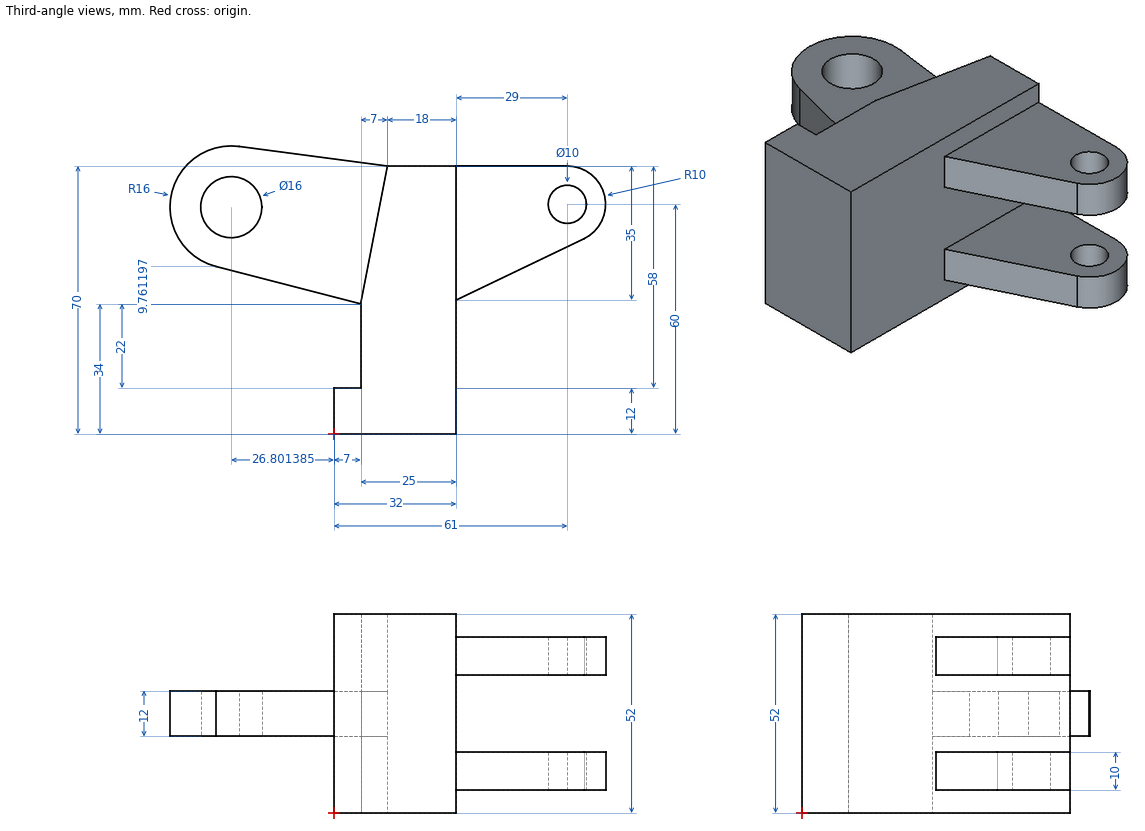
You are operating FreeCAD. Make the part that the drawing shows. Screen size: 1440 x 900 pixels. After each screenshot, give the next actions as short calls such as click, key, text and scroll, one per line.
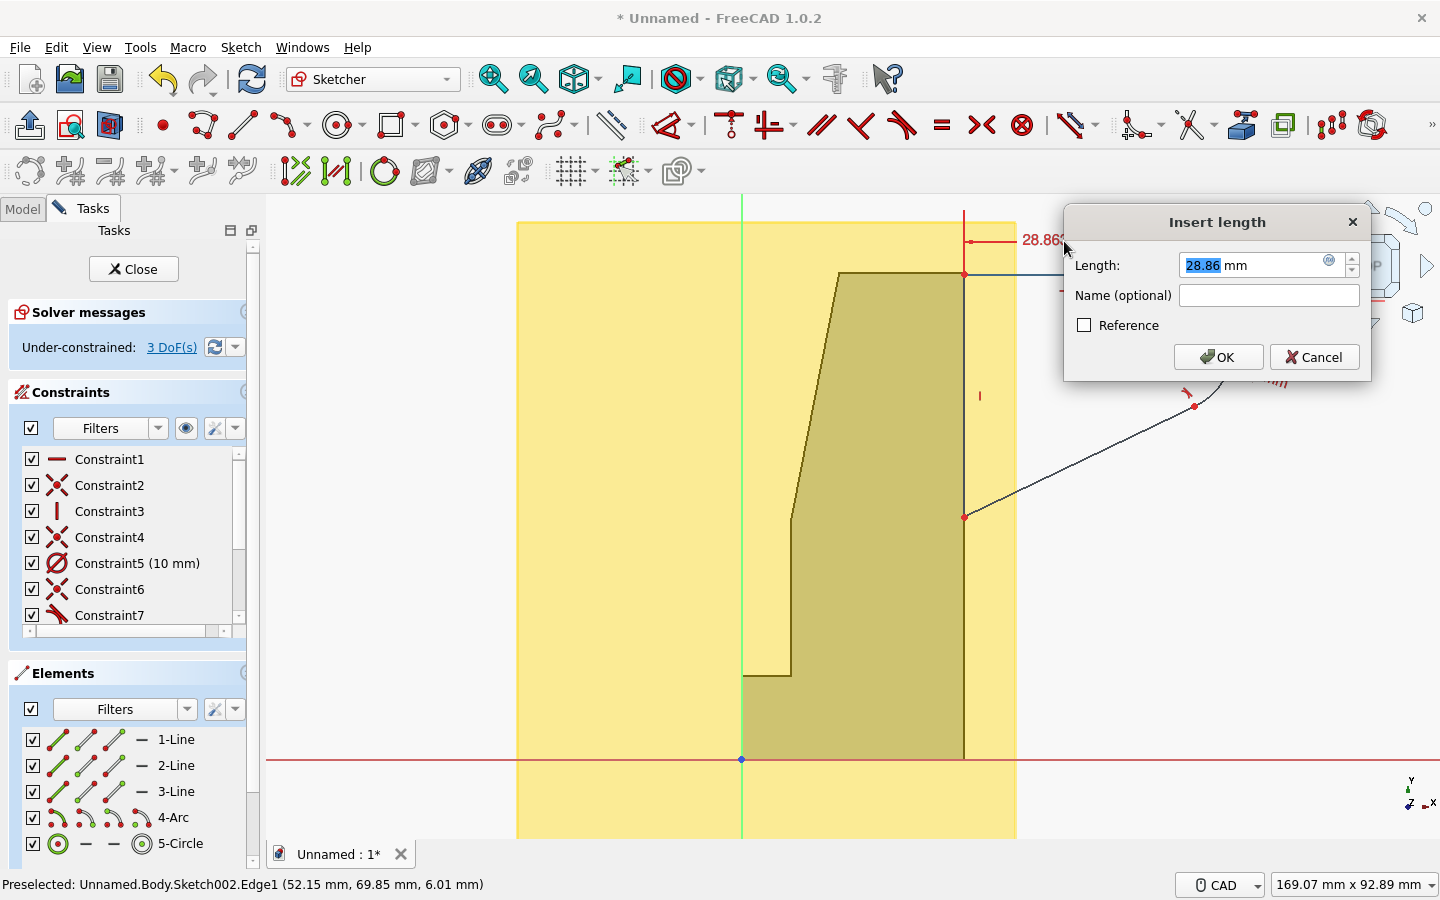
text(29)
key(Return)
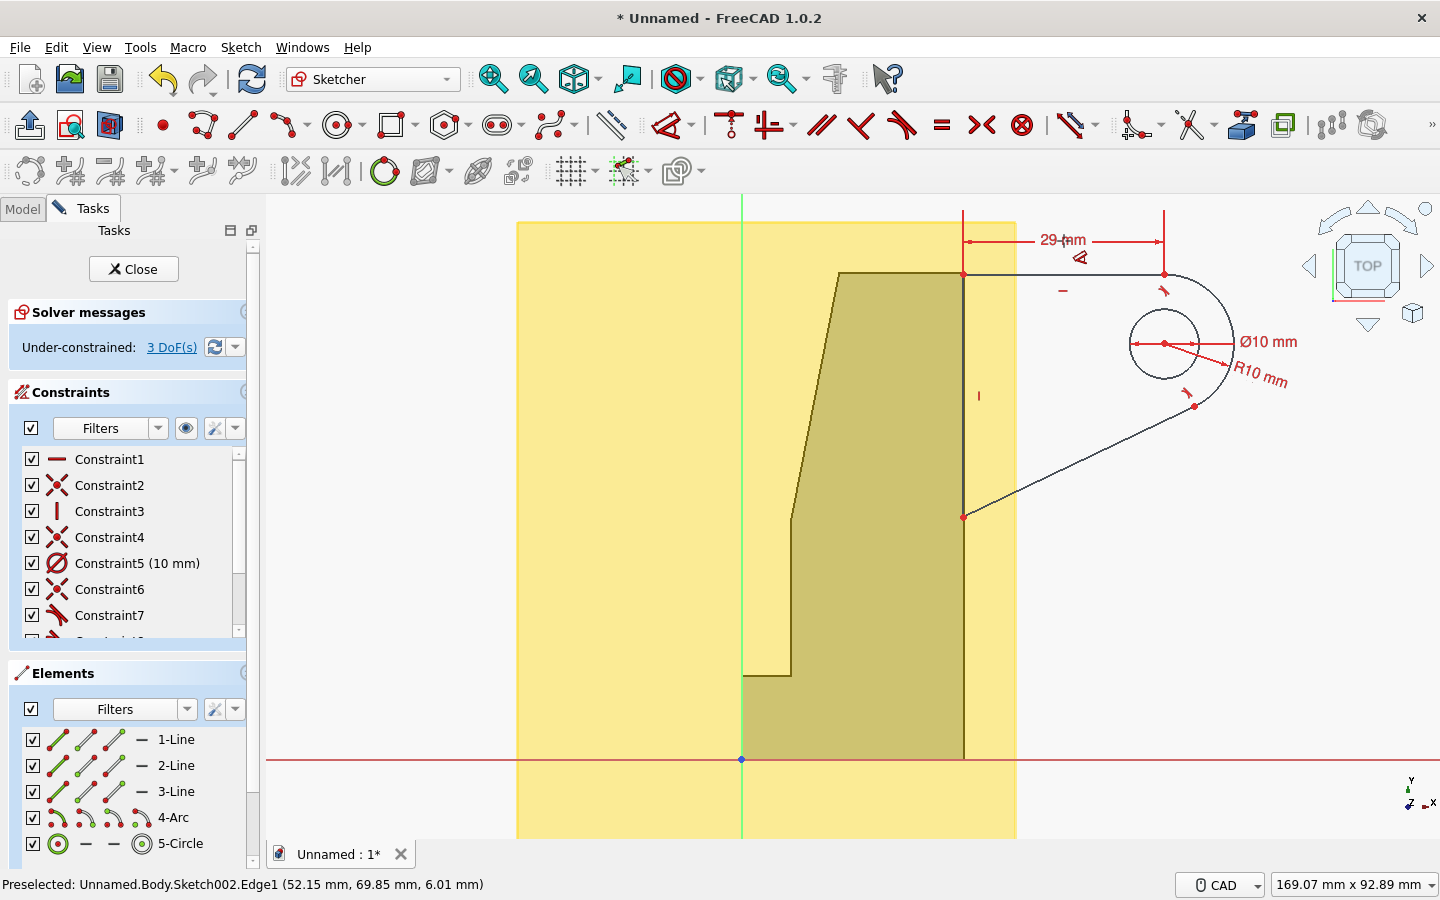
click(963, 347)
click(929, 396)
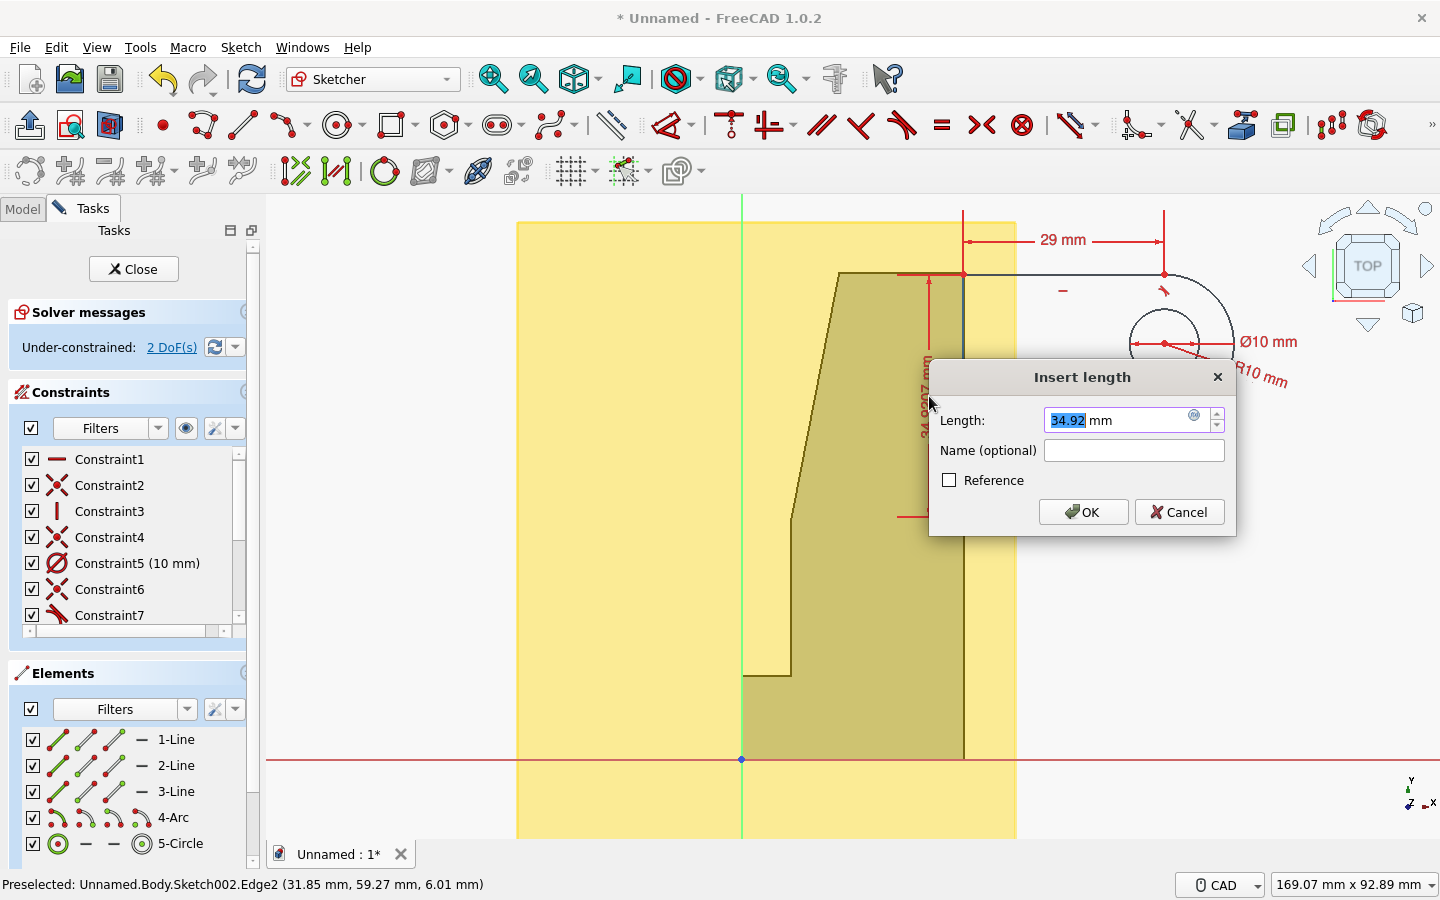
text(35)
key(Return)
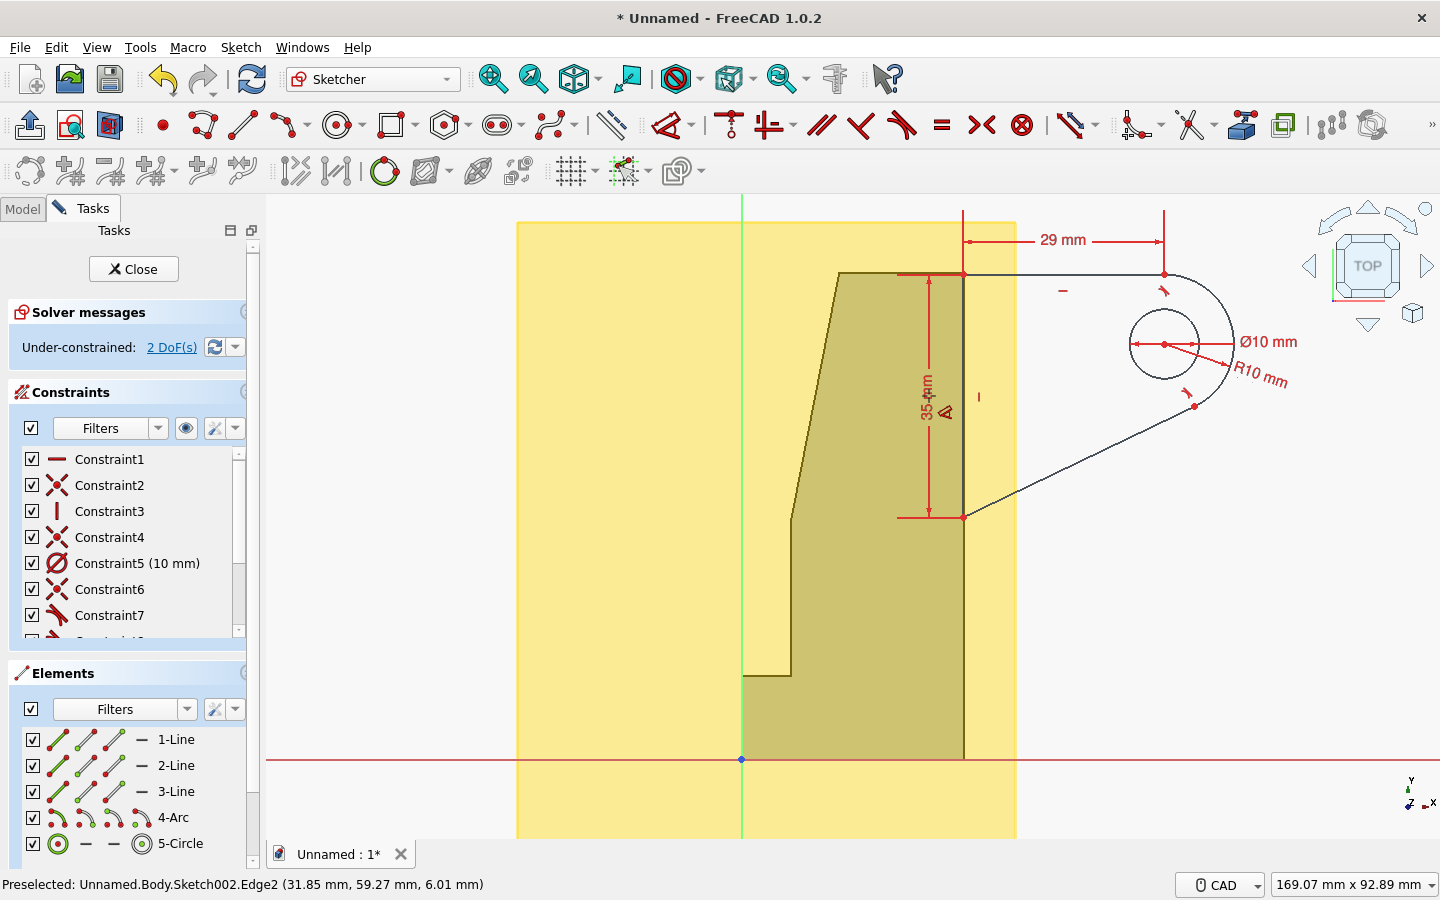
click(1164, 344)
click(953, 794)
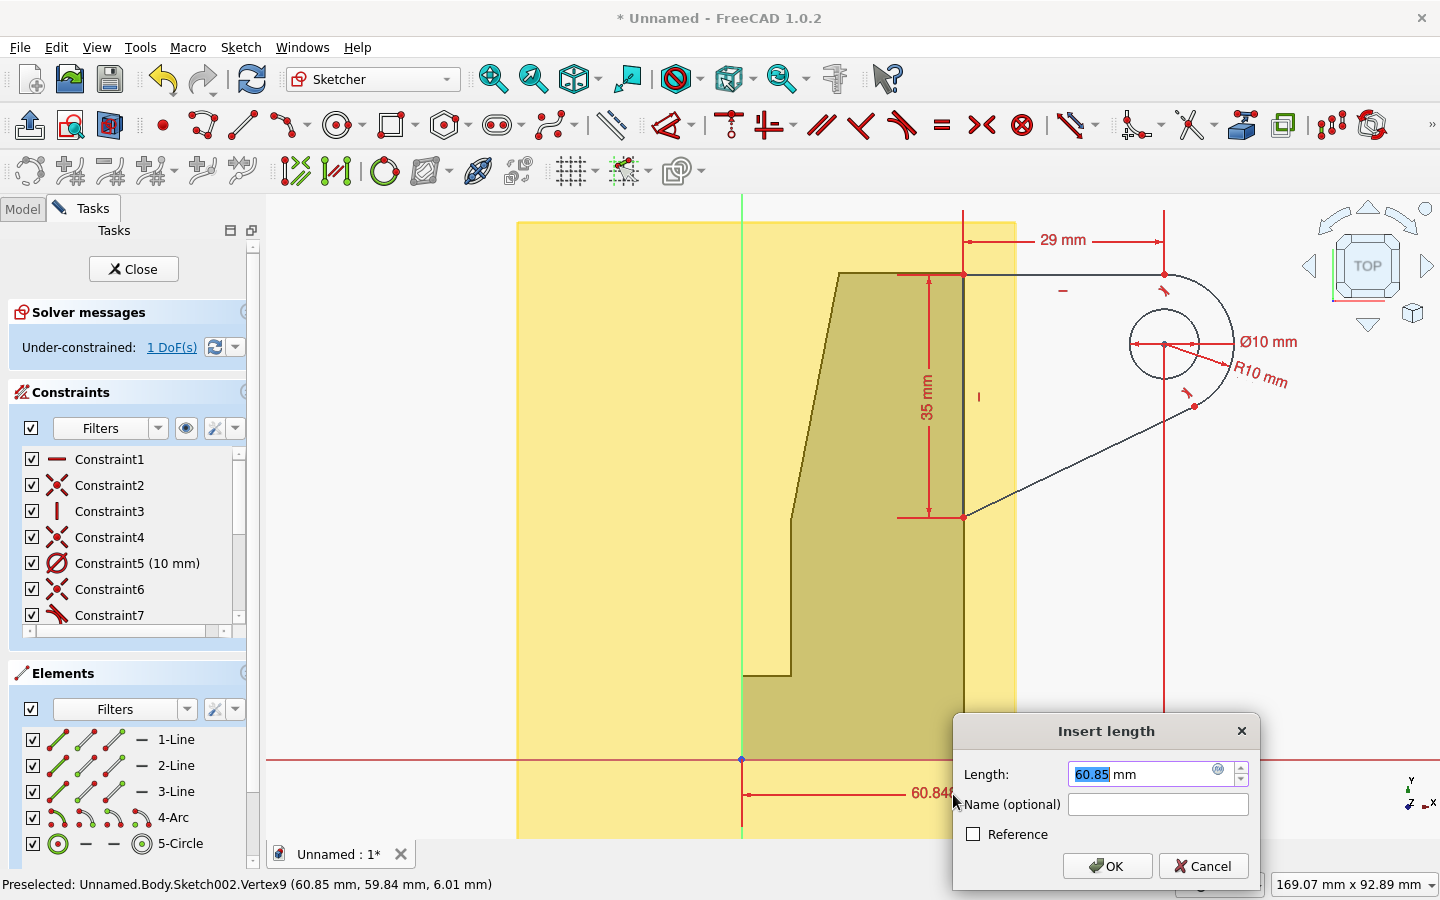
text(61)
key(Return)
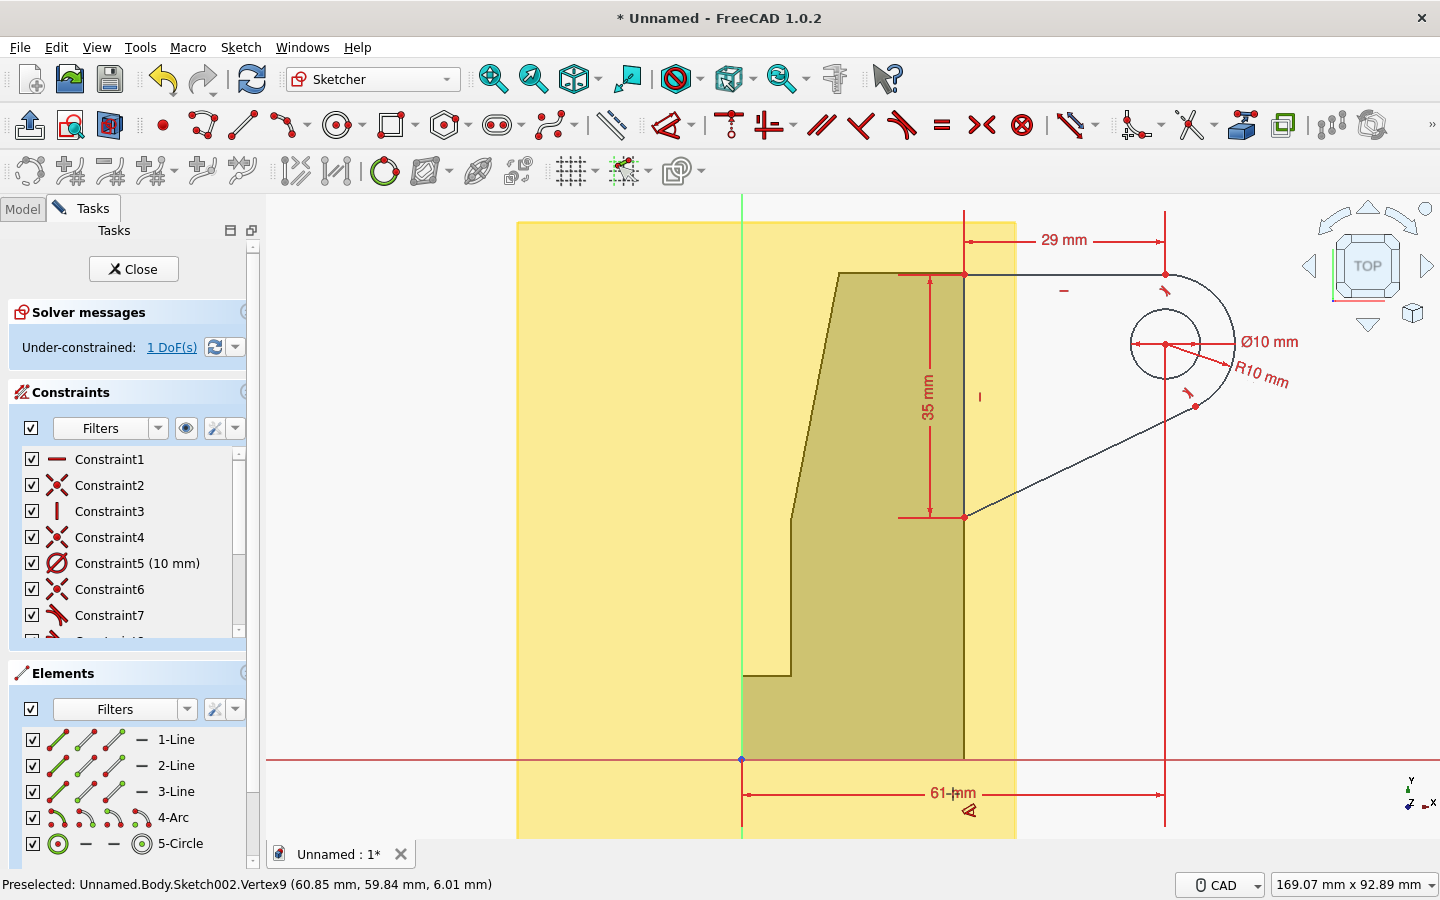
click(1165, 344)
click(708, 552)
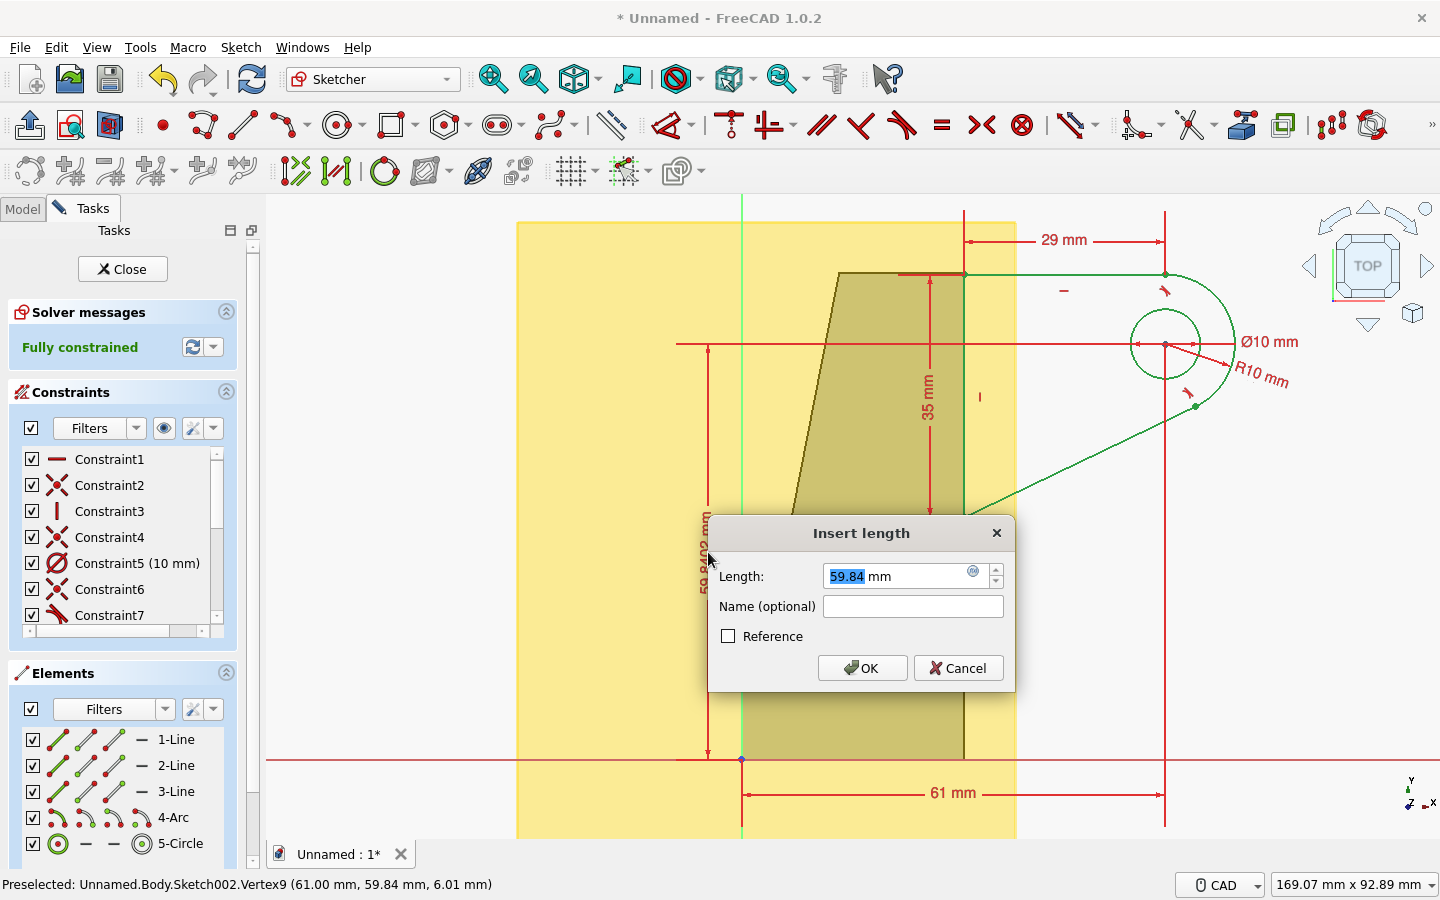
text(60)
key(Return)
key(Escape)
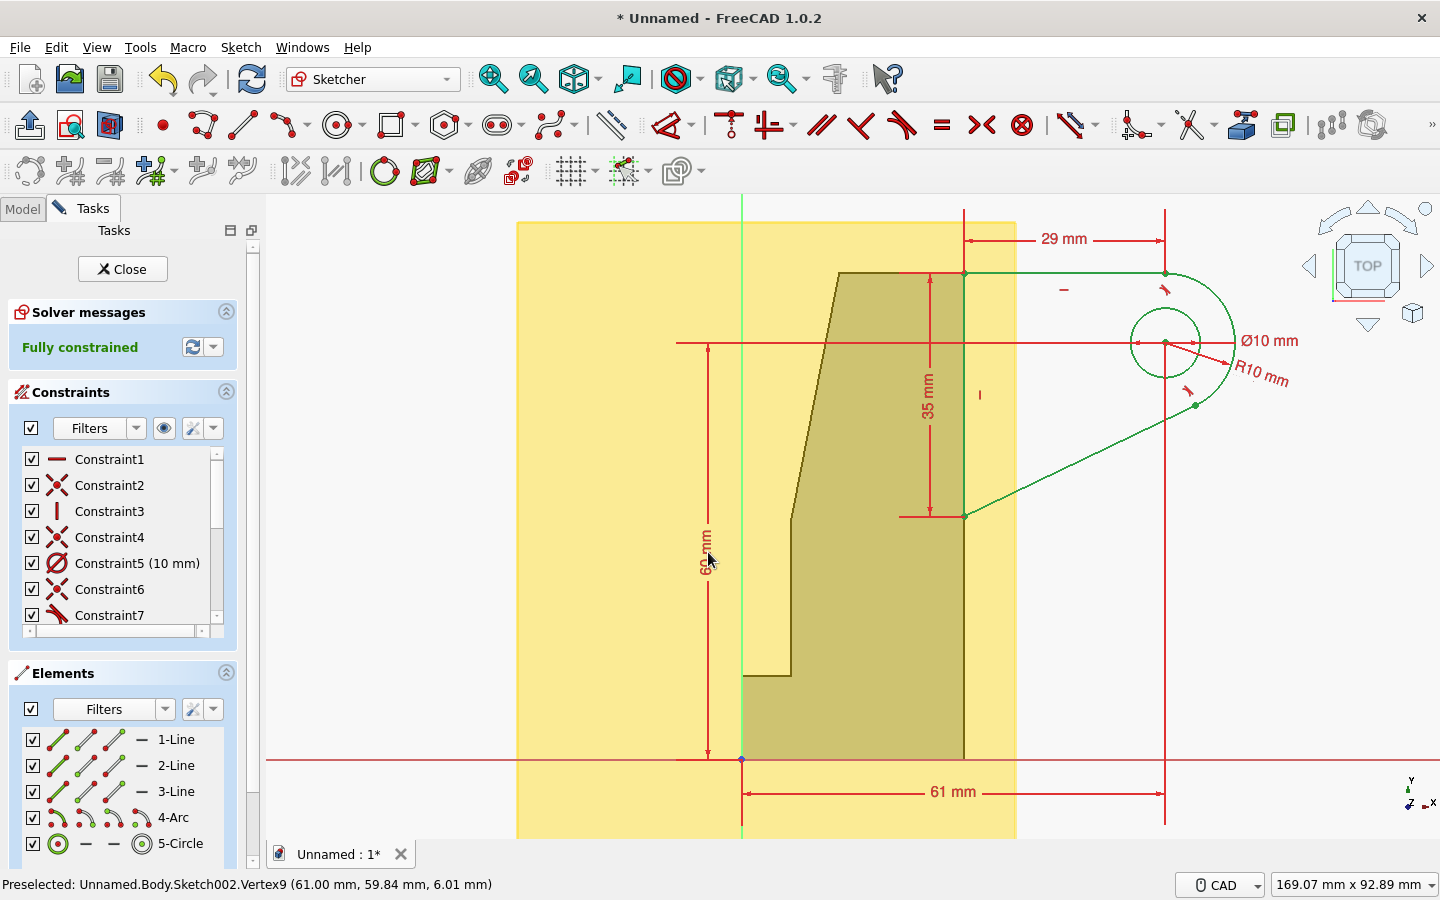
click(123, 269)